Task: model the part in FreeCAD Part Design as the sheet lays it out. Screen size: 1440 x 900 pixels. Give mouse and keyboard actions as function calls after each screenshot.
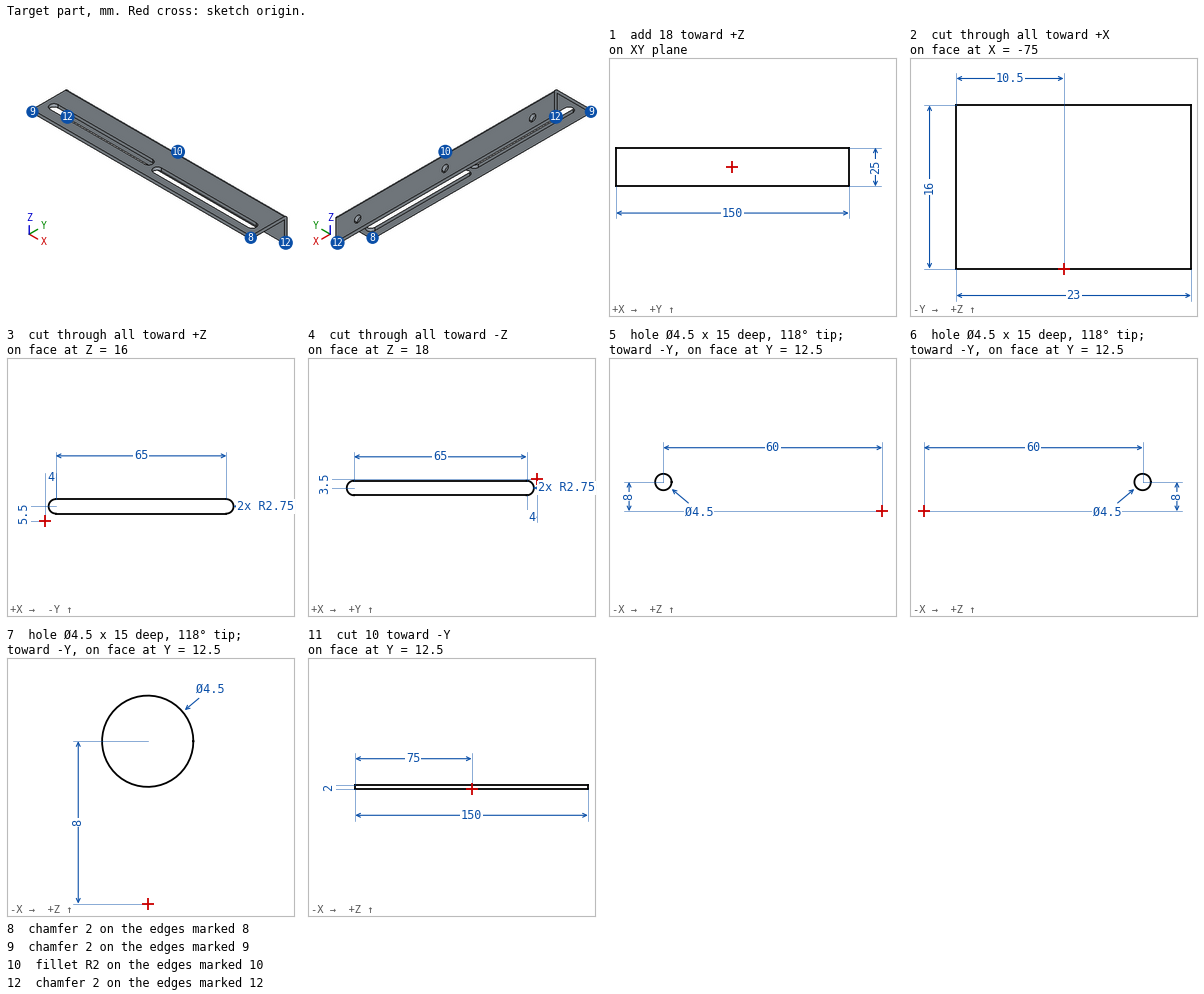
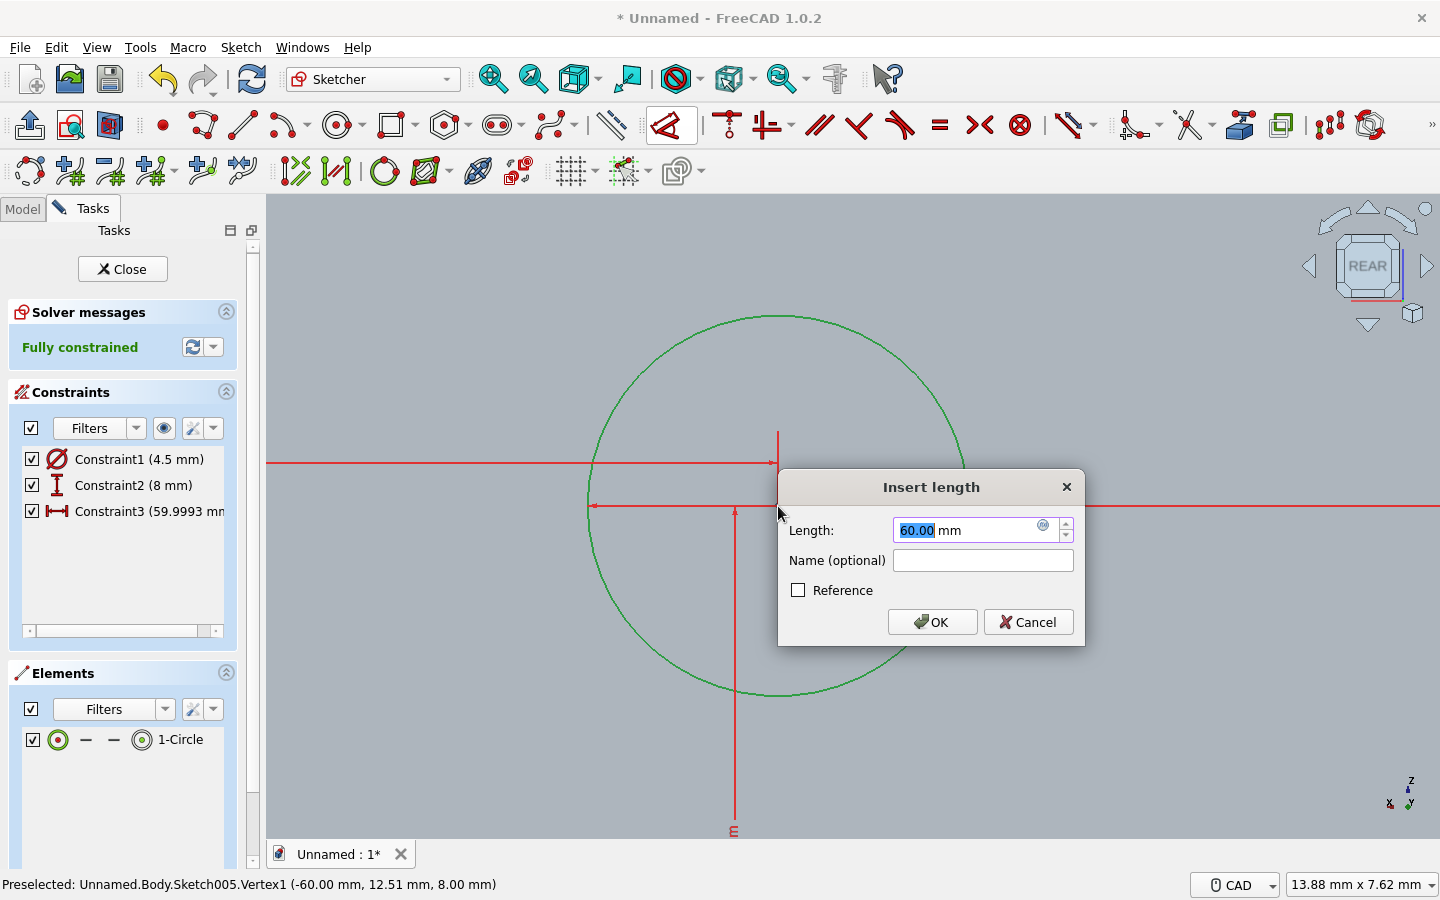
text(60)
key(Return)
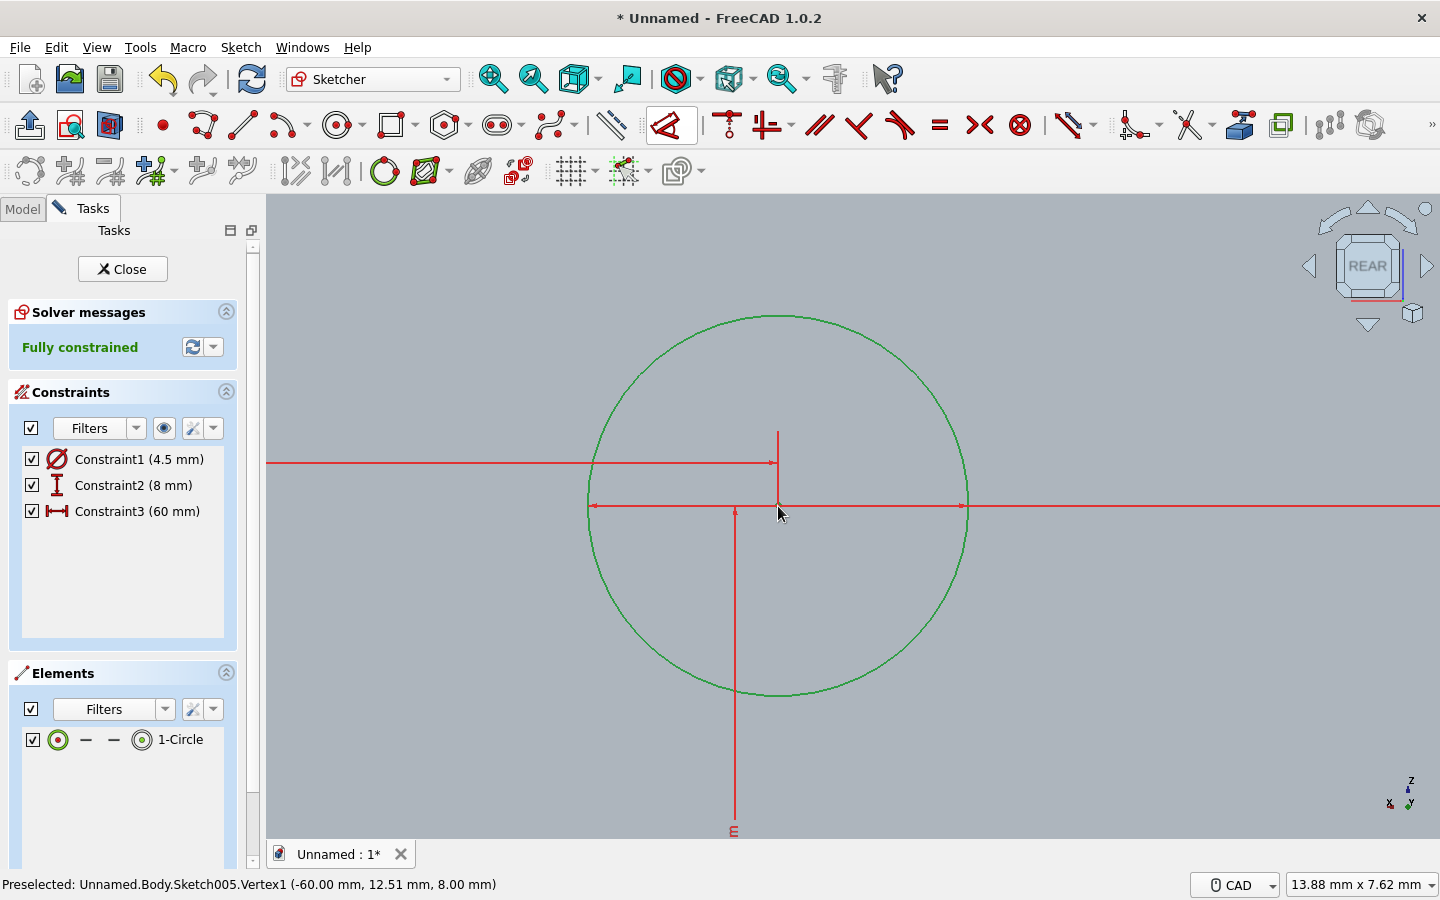
click(123, 269)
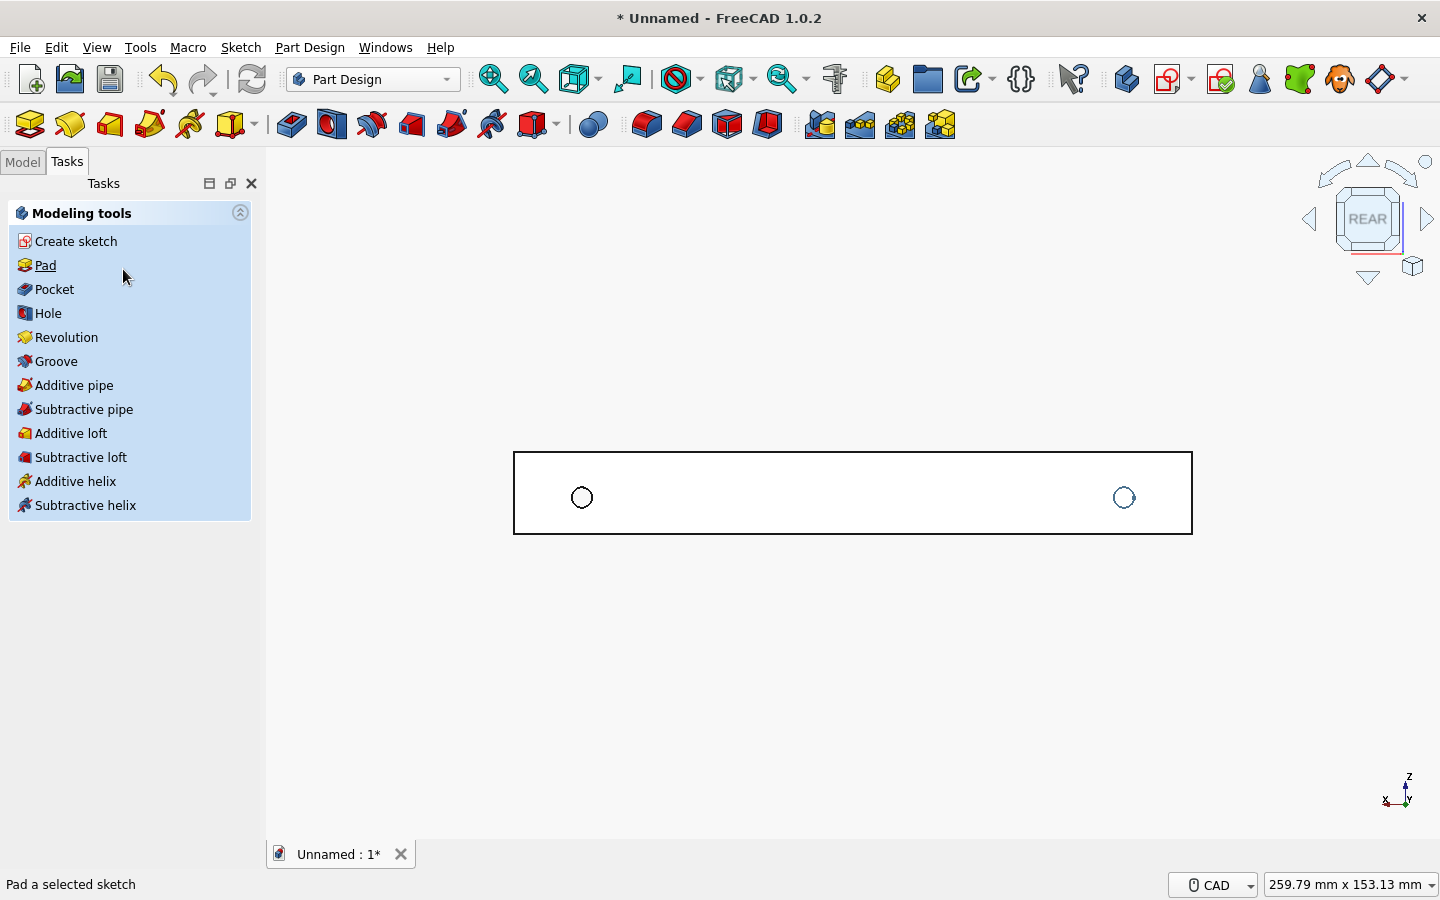
click(332, 124)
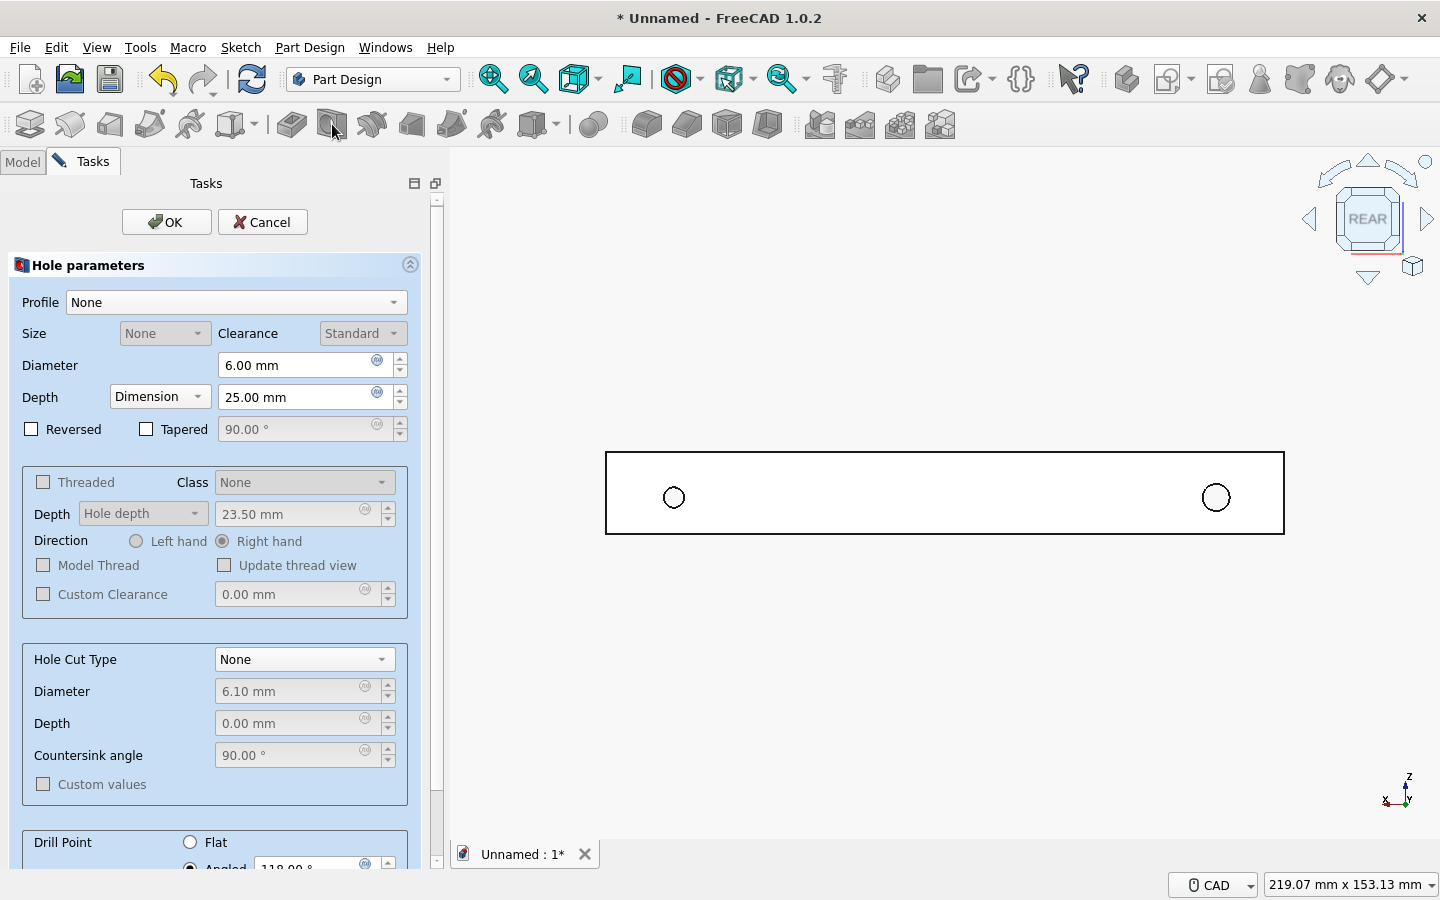
triple_click(305, 365)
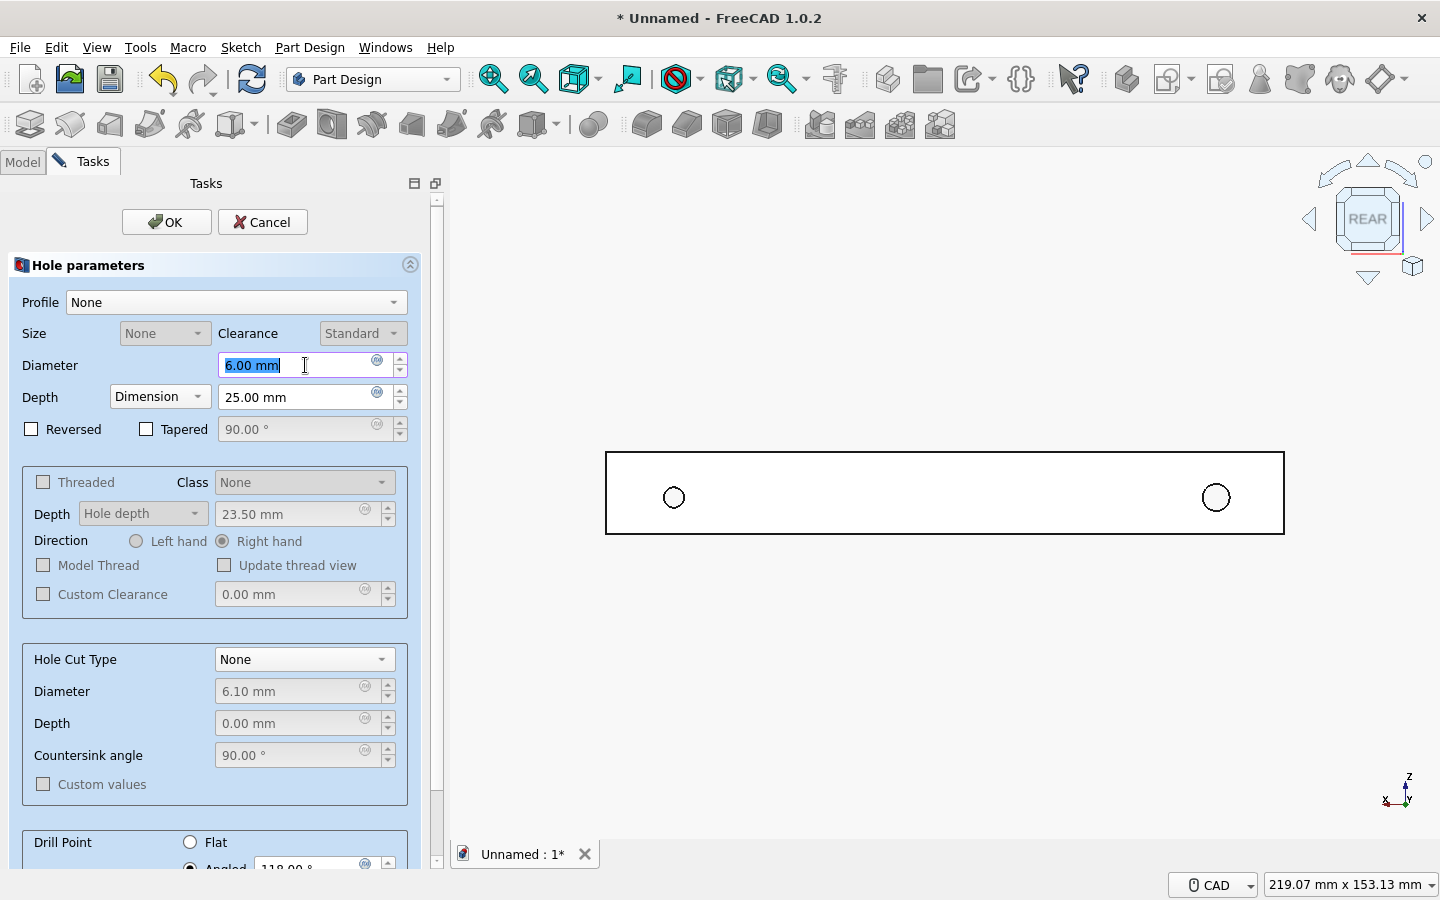
text(4.5)
key(Tab)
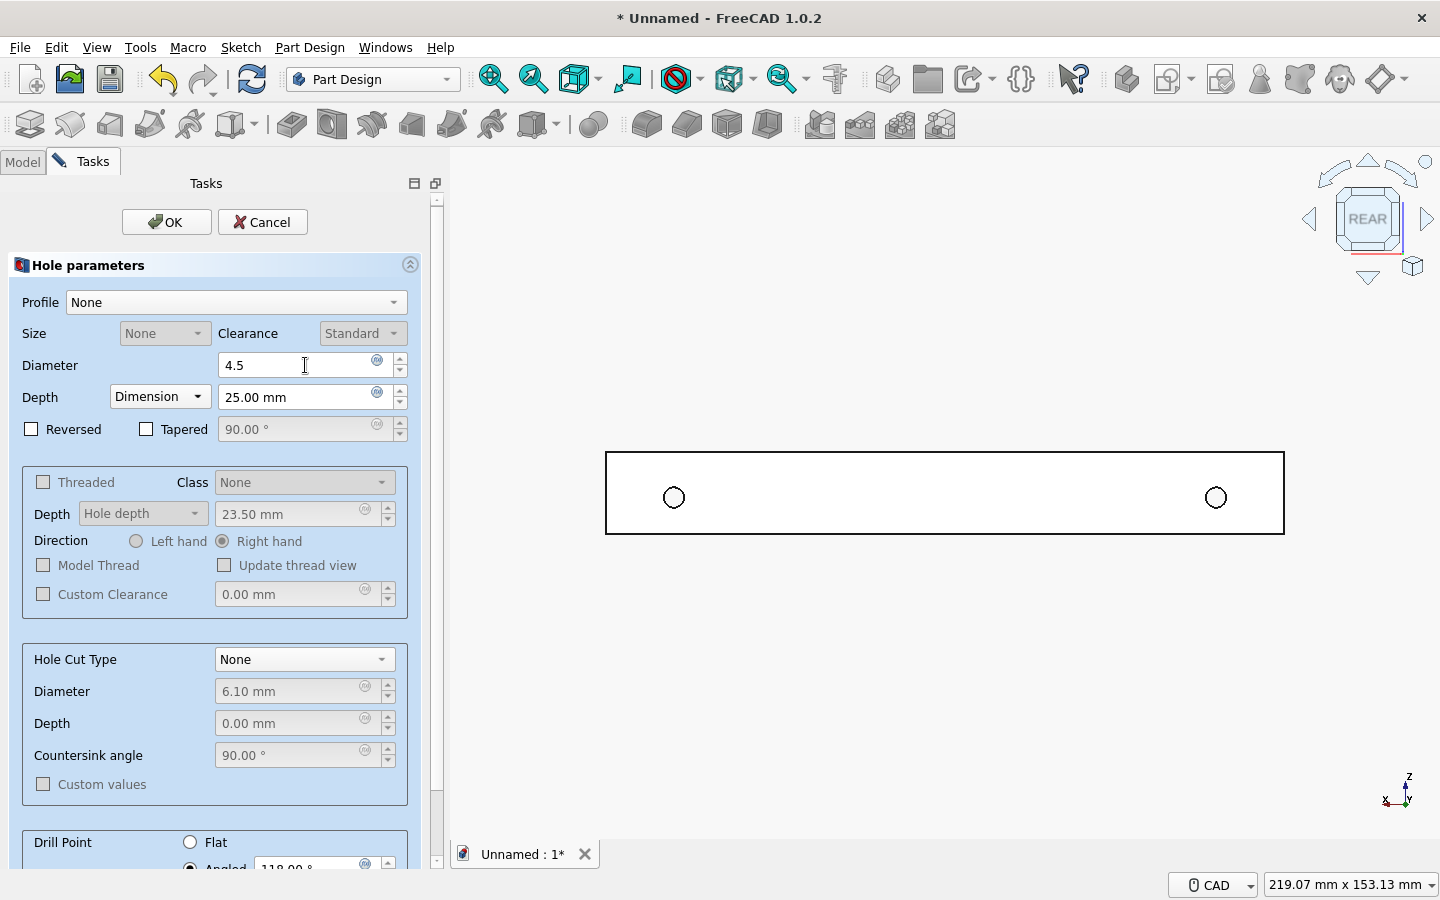
triple_click(305, 397)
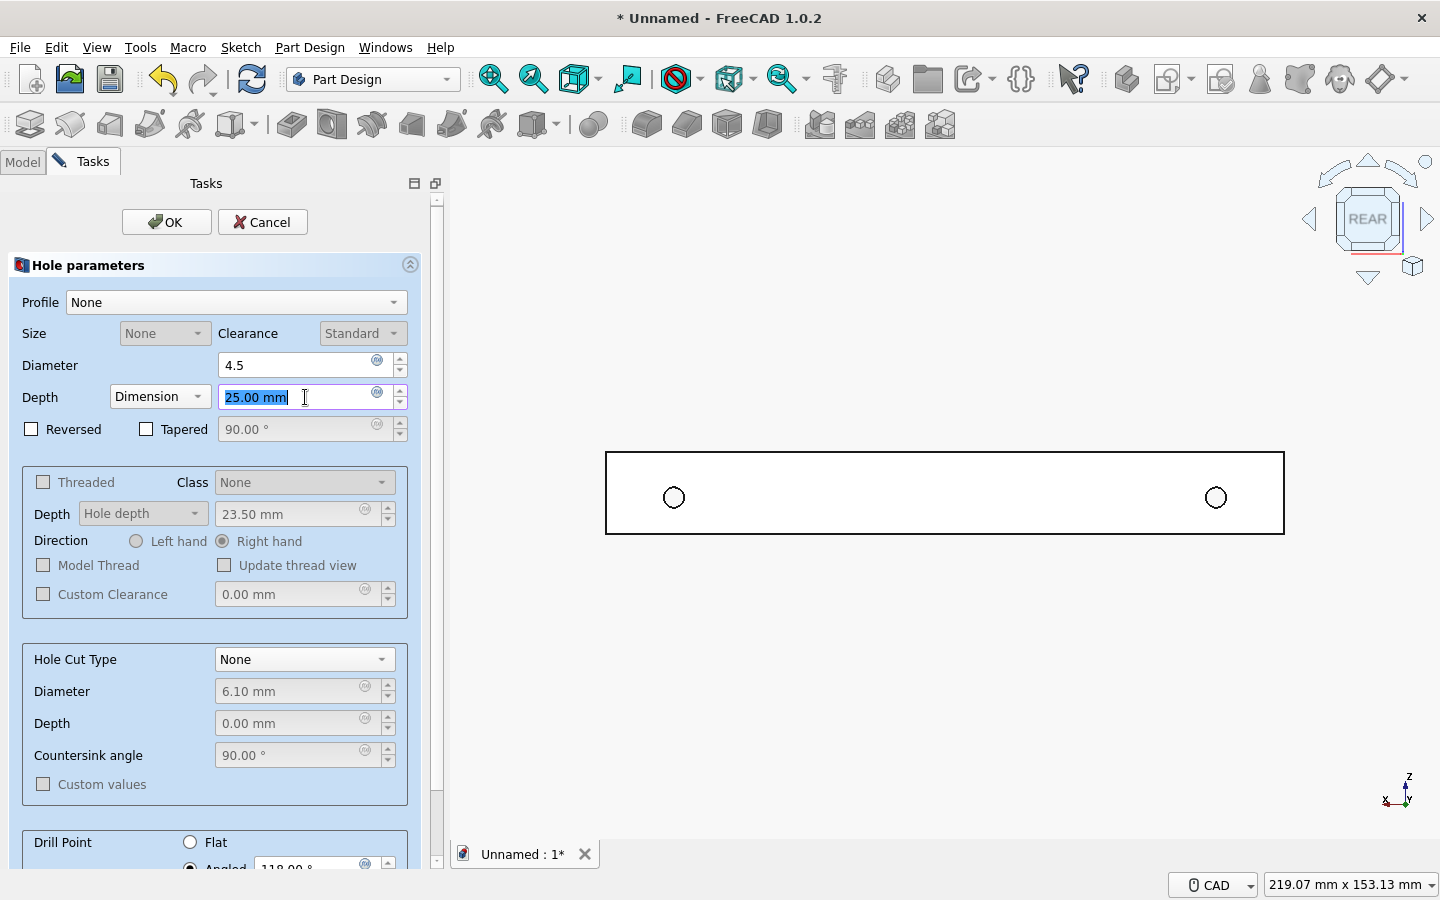
text(15)
key(Tab)